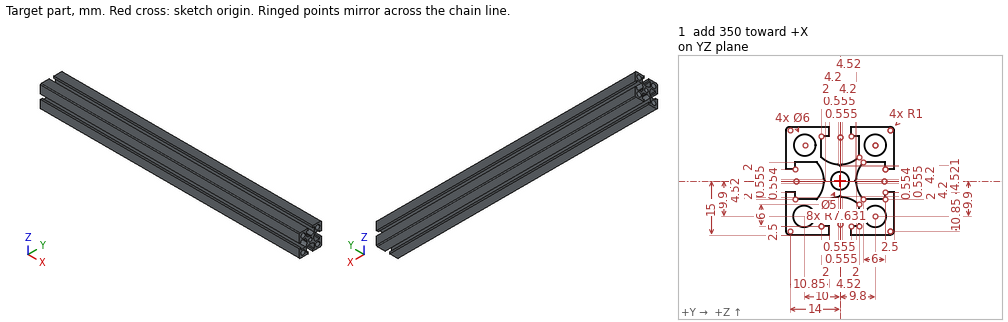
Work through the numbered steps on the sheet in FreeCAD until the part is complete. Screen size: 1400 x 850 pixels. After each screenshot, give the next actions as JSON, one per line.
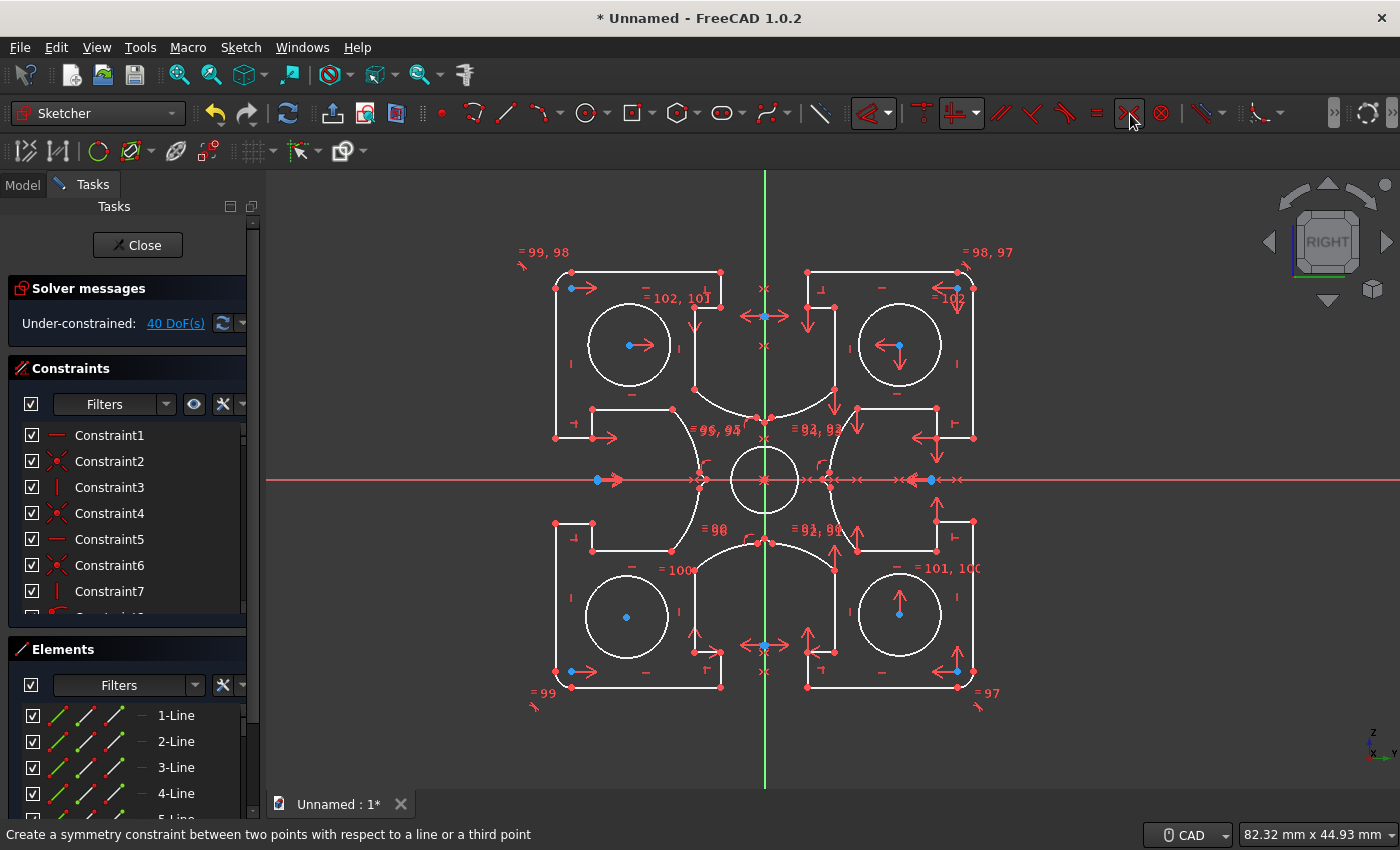
{"action": "left_click", "coordinate": [937, 551]}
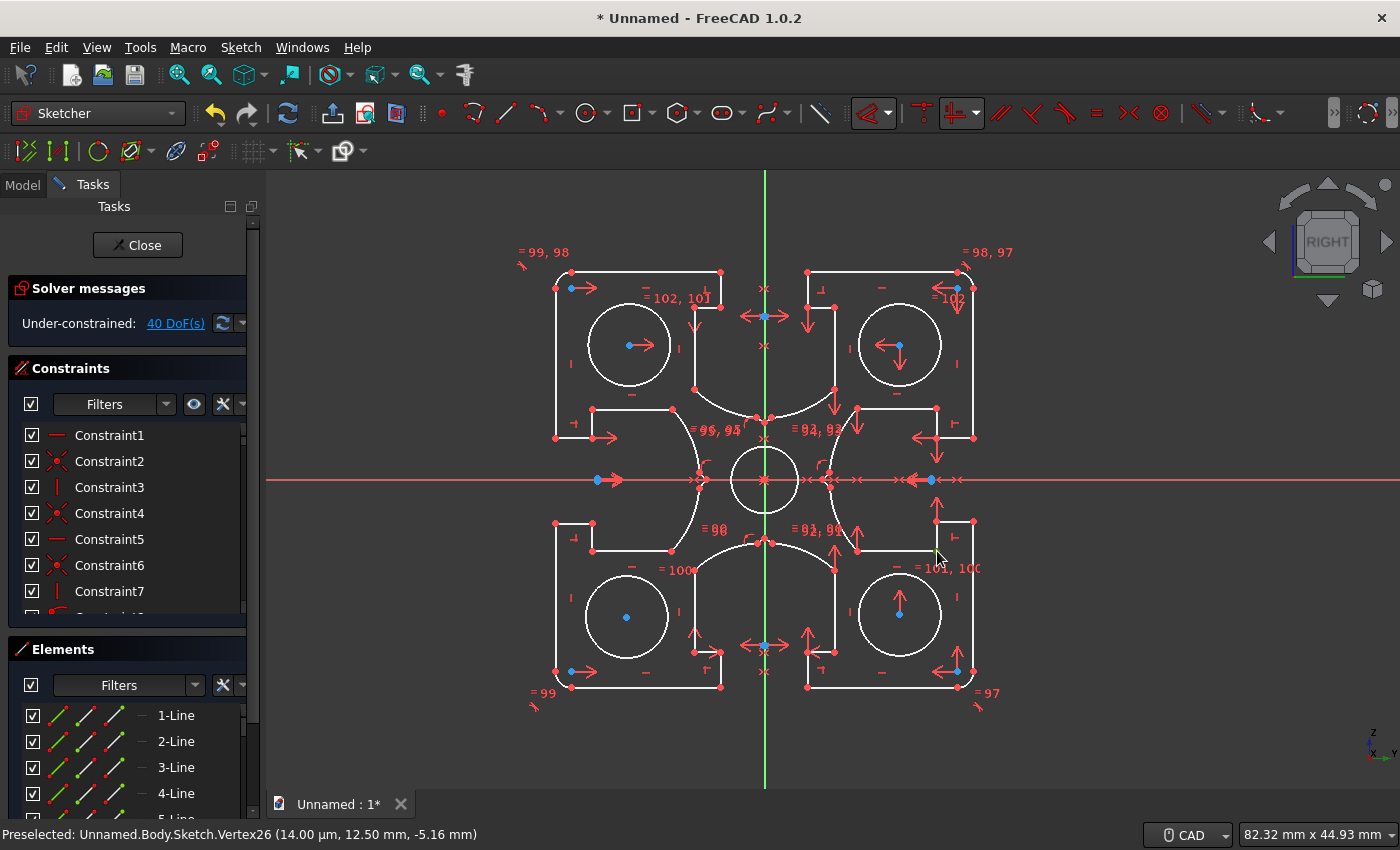
{"action": "left_click", "coordinate": [592, 551]}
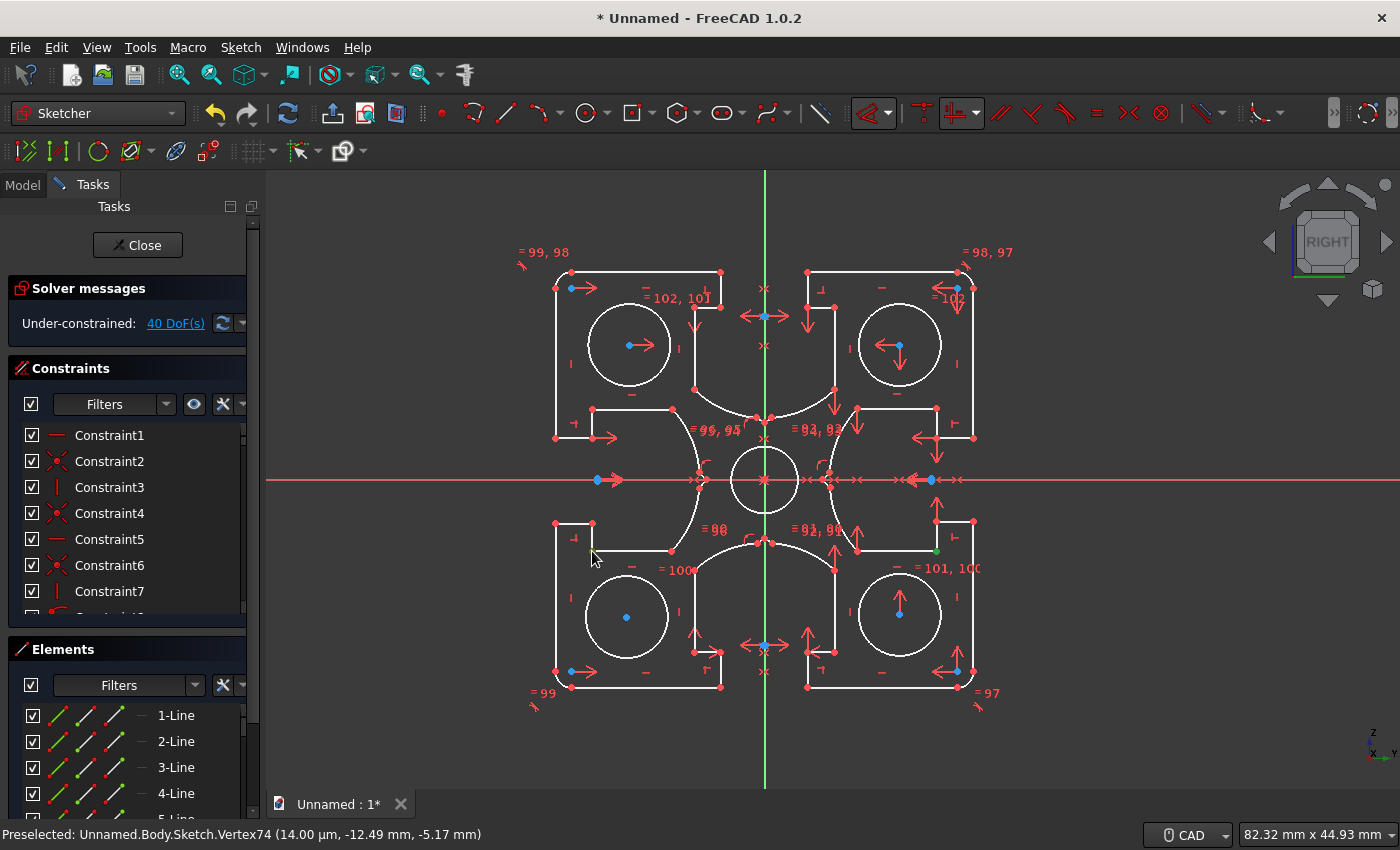
{"action": "left_click", "coordinate": [765, 721]}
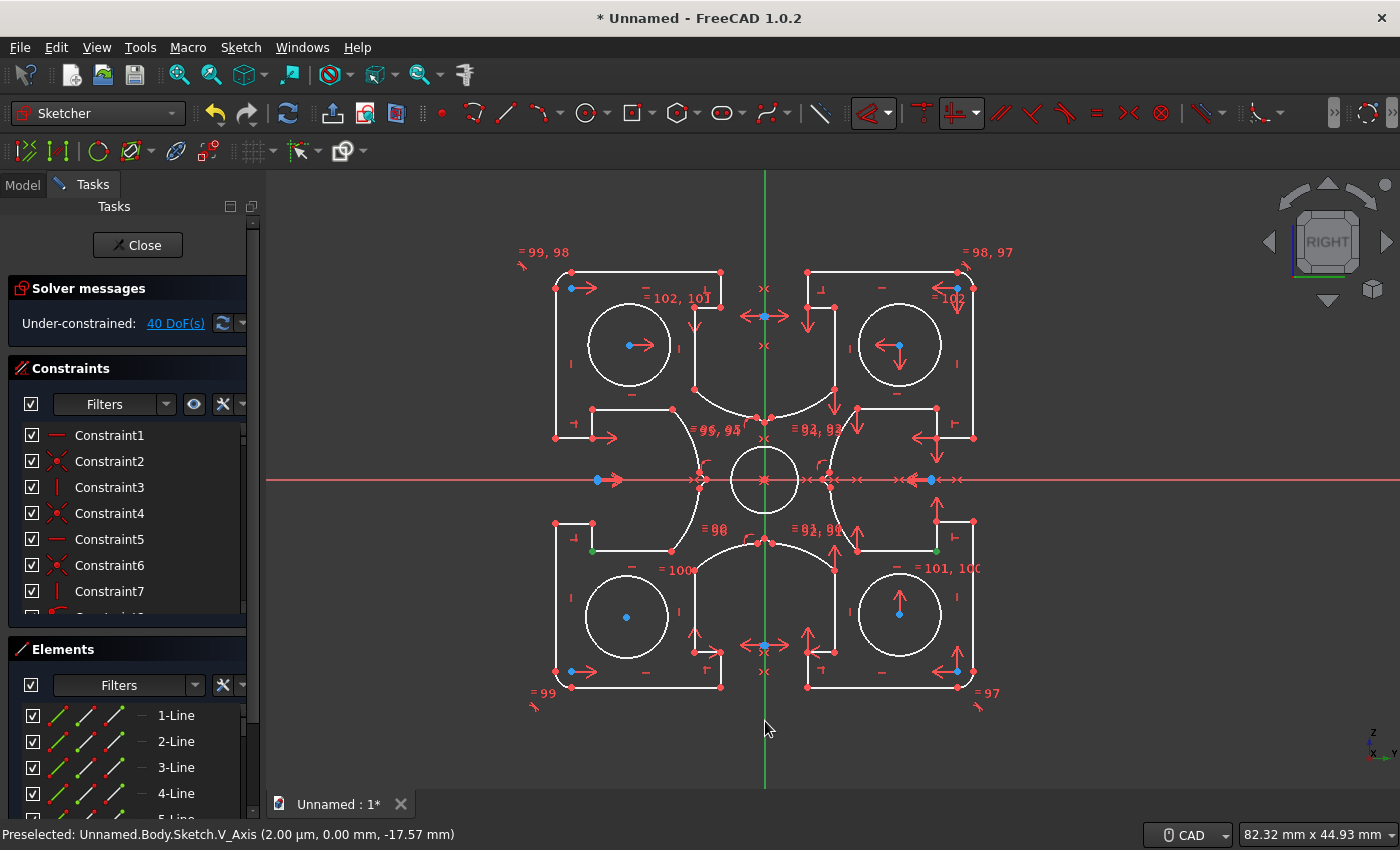
{"action": "key", "text": "s"}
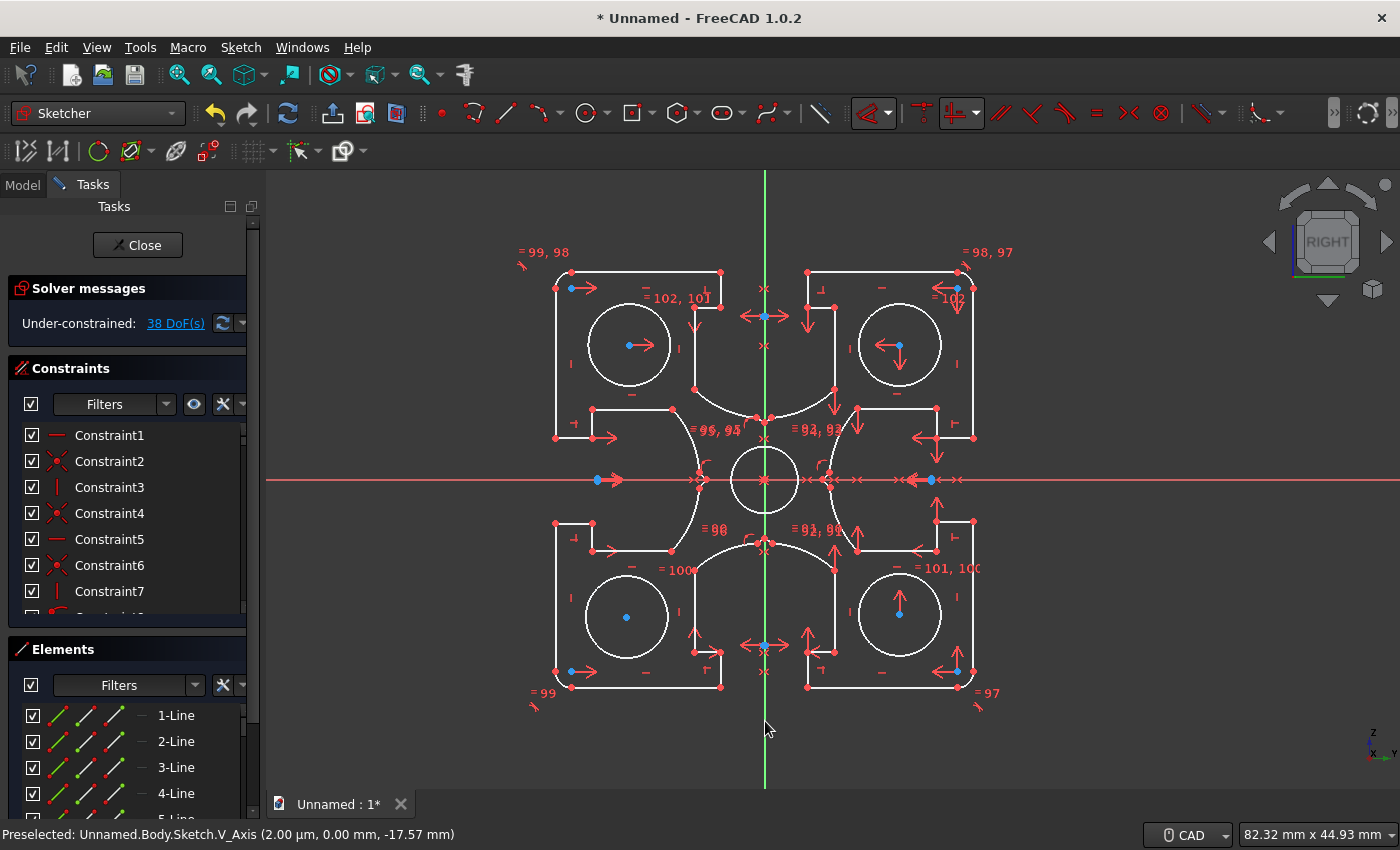
{"action": "key", "text": "d"}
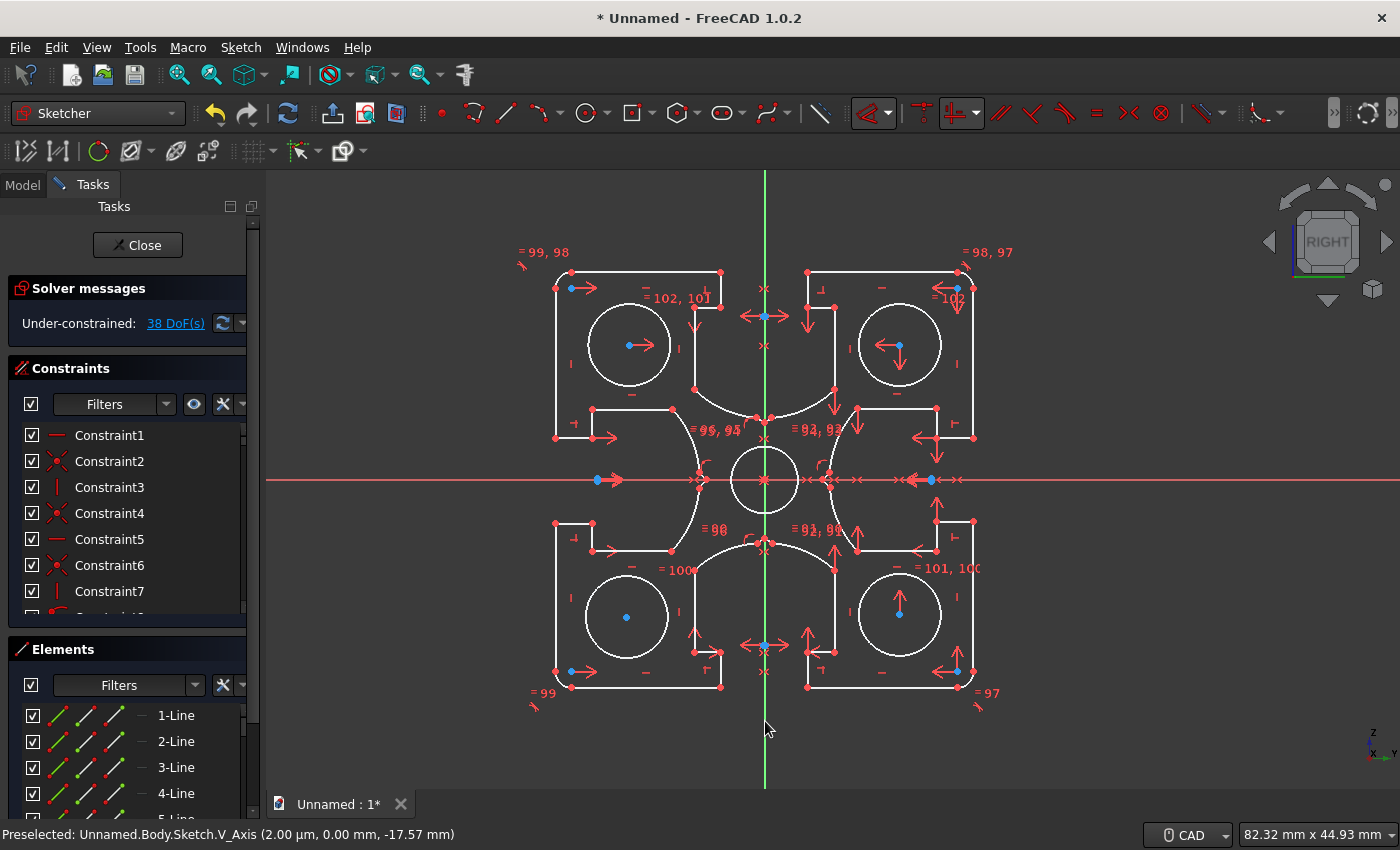
{"action": "left_click", "coordinate": [737, 547]}
{"action": "left_click", "coordinate": [729, 516]}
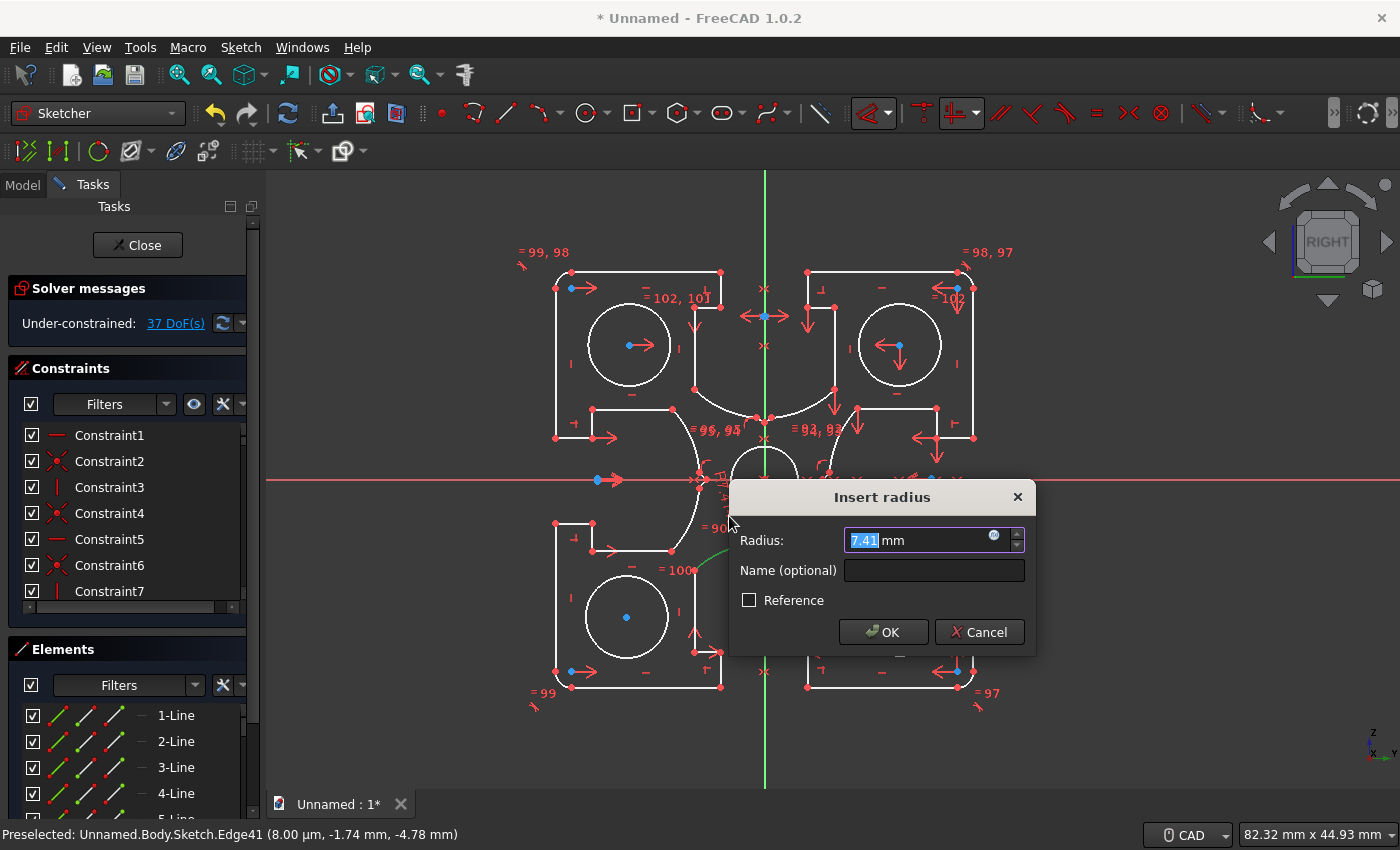
{"action": "type", "text": "7.631"}
{"action": "key", "text": "Return"}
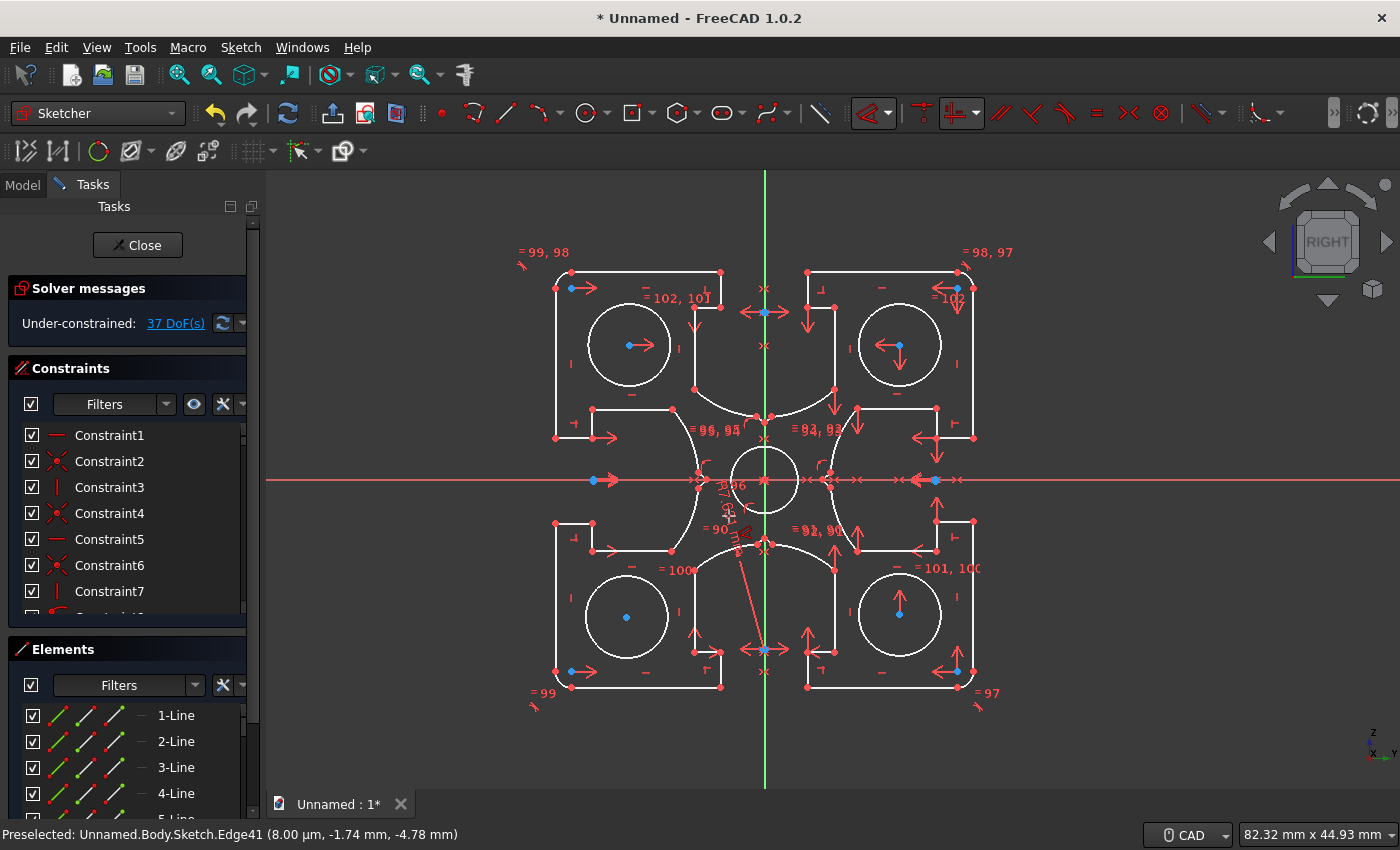
{"action": "scroll", "coordinate": [969, 683], "scroll_direction": "up", "scroll_amount": 6}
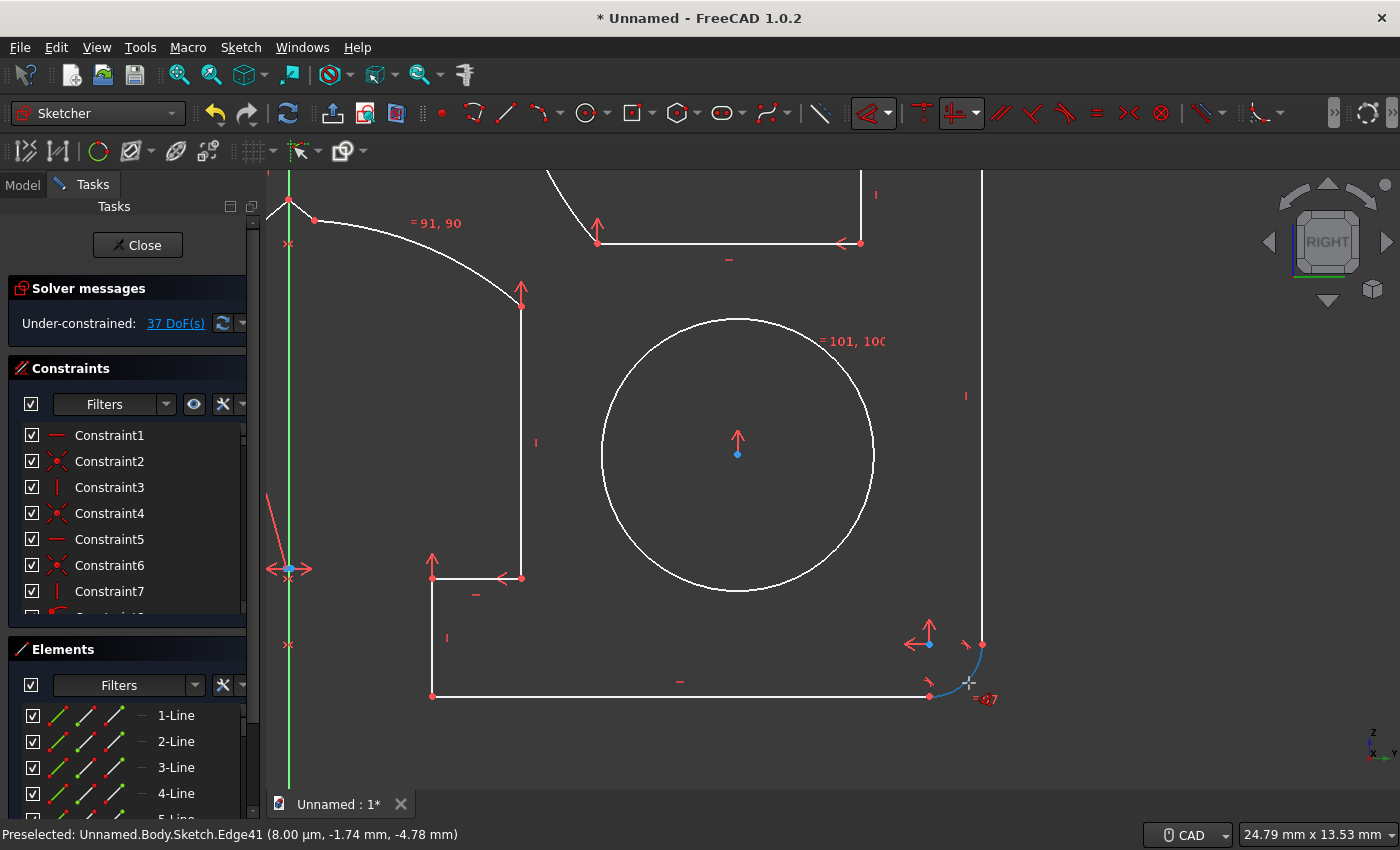
{"action": "left_click", "coordinate": [967, 682]}
{"action": "left_click", "coordinate": [990, 705]}